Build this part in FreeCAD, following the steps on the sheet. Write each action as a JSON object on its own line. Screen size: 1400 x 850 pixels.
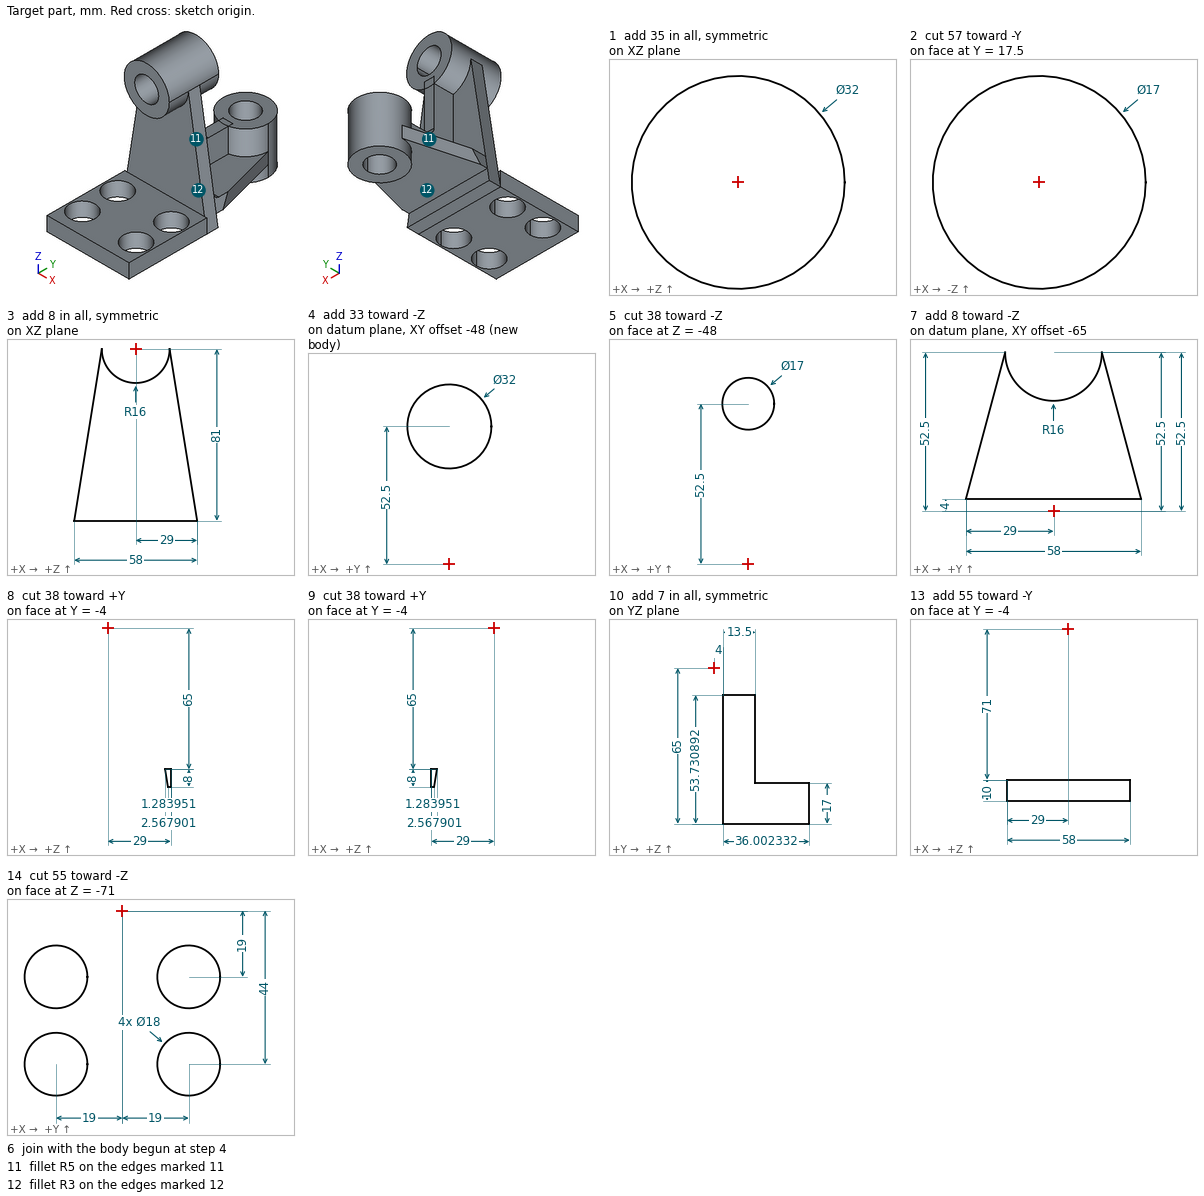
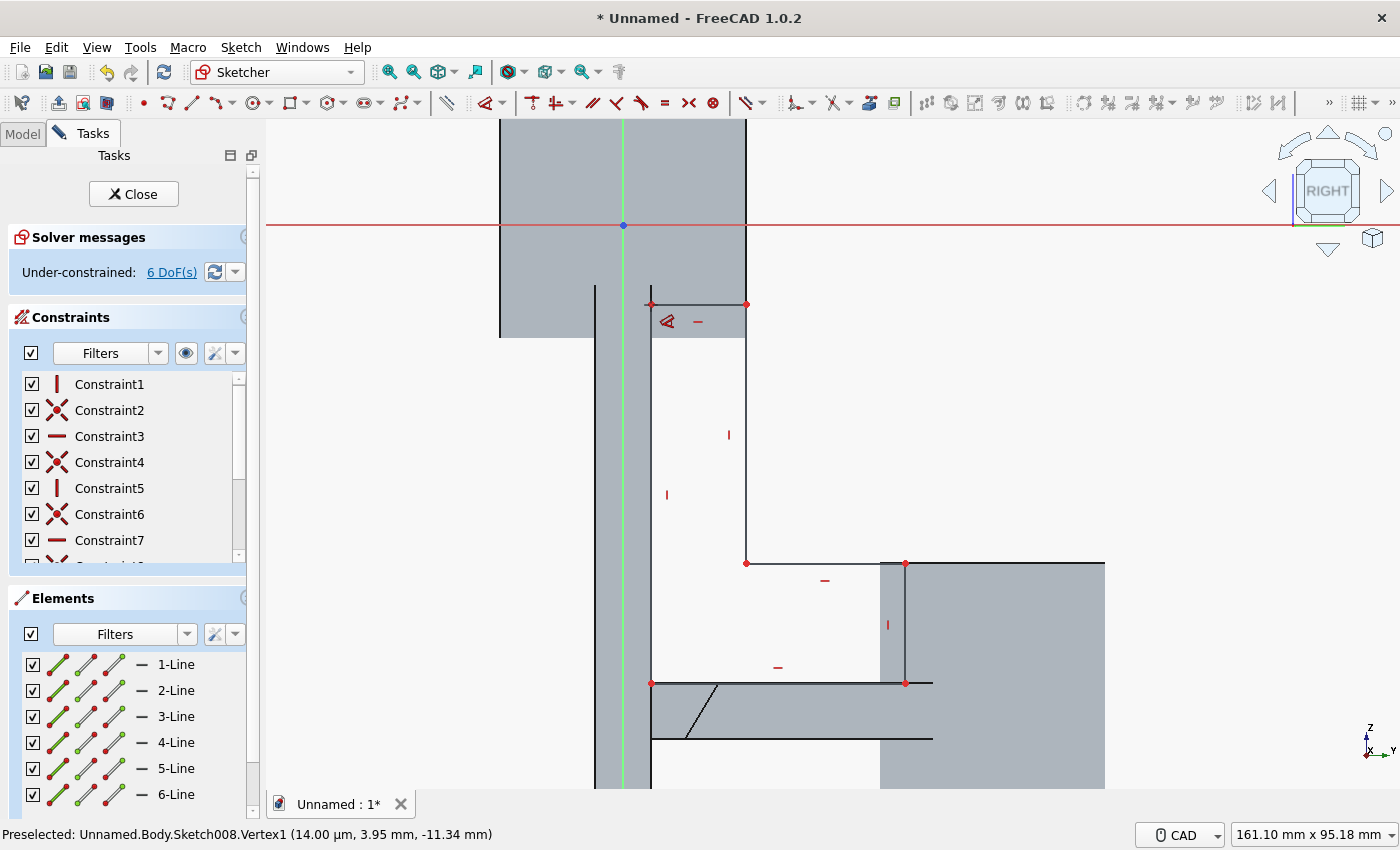
{"action": "left_click", "coordinate": [905, 648]}
{"action": "left_click", "coordinate": [939, 624]}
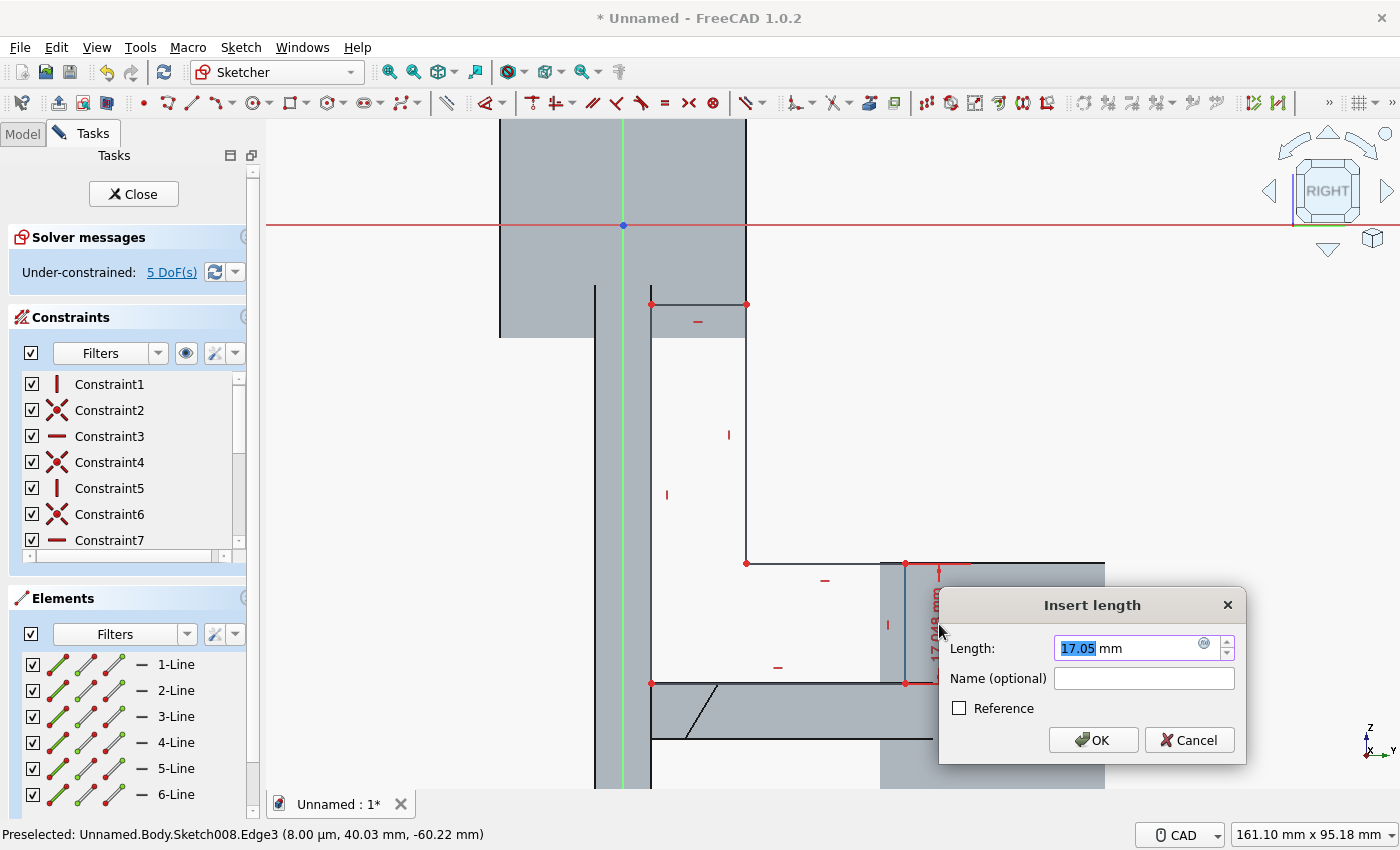
{"action": "type", "text": "17"}
{"action": "key", "text": "Return"}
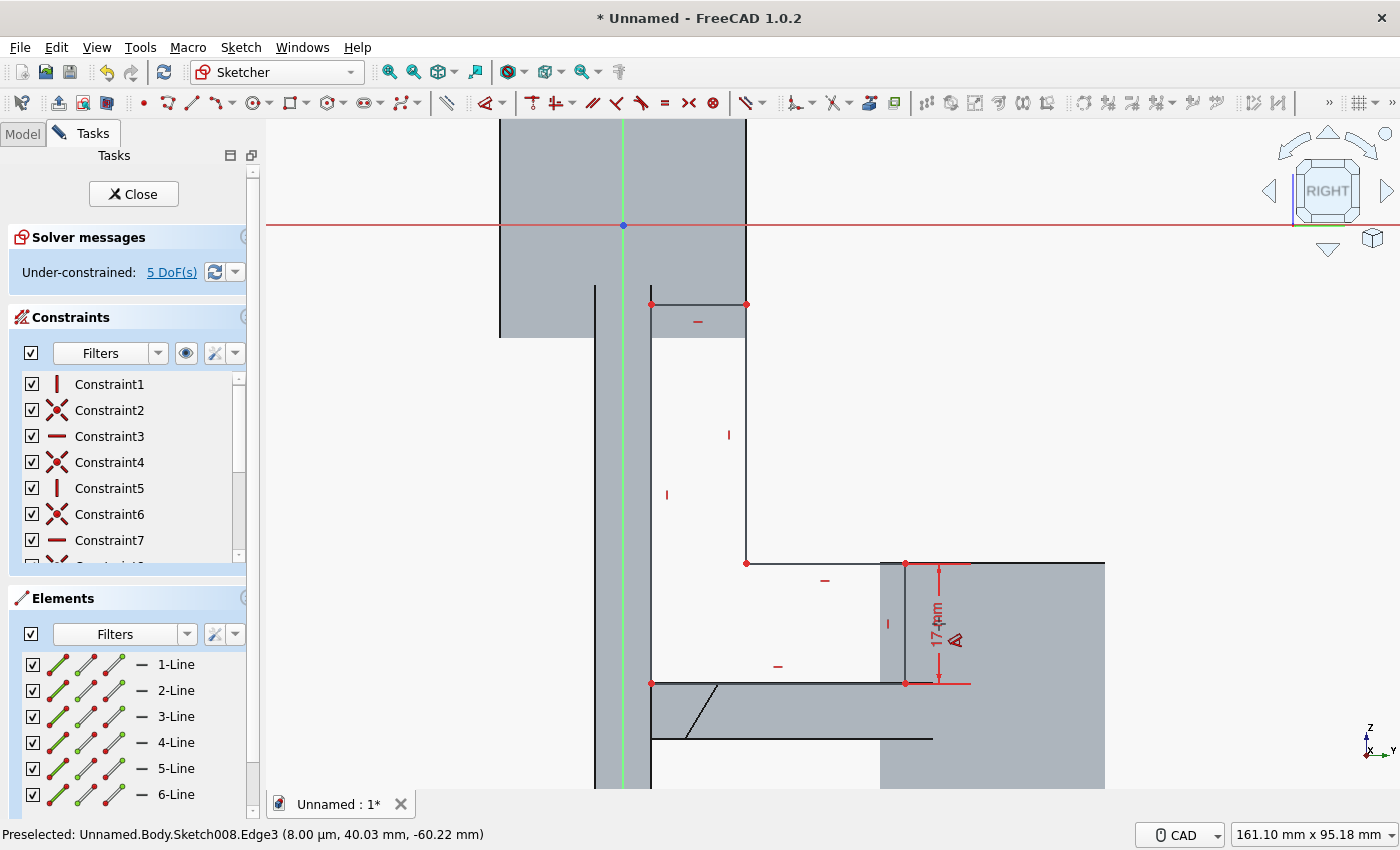
{"action": "scroll", "coordinate": [651, 305], "scroll_direction": "up", "scroll_amount": 2}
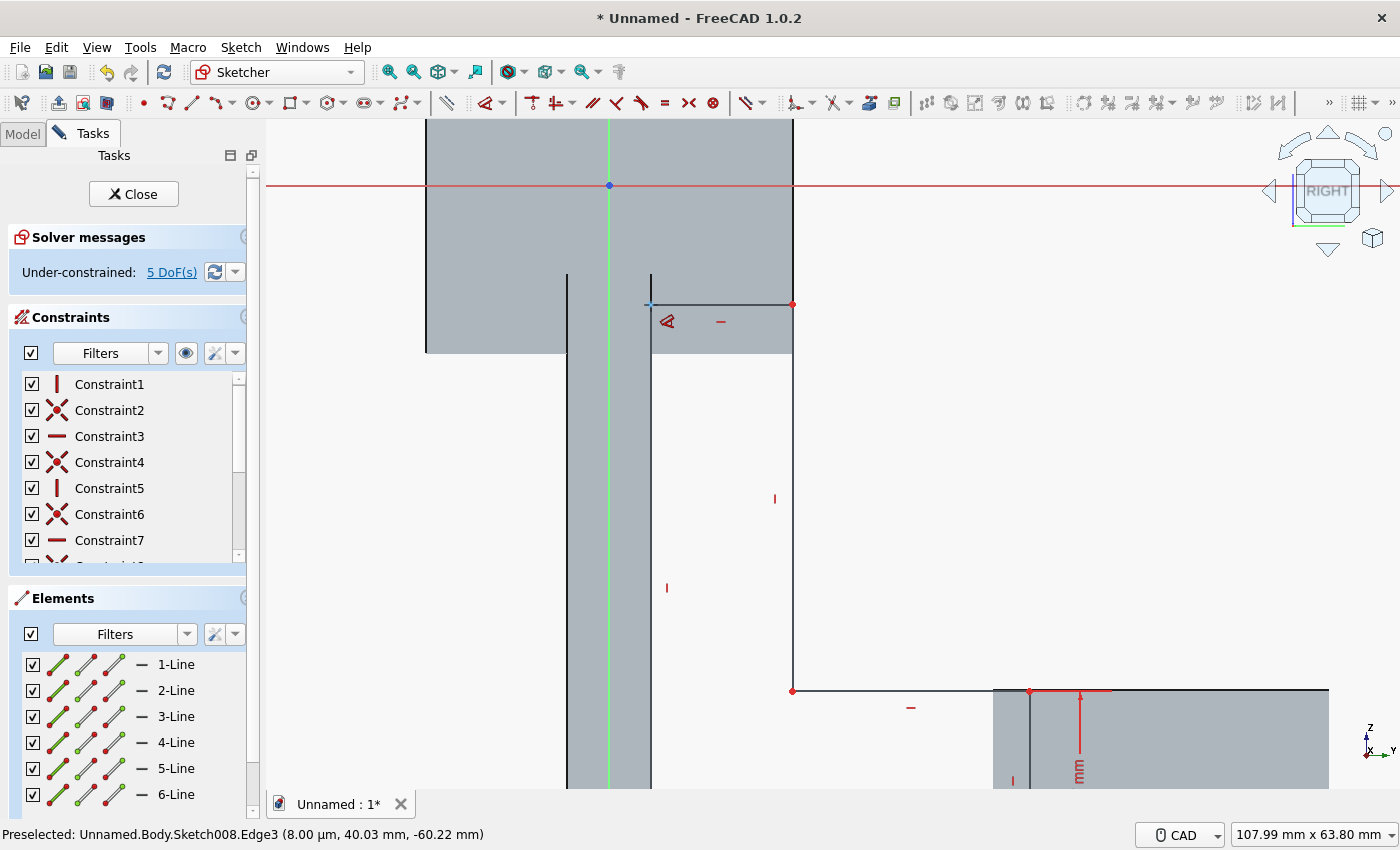
{"action": "left_click", "coordinate": [651, 305]}
{"action": "left_click", "coordinate": [630, 152]}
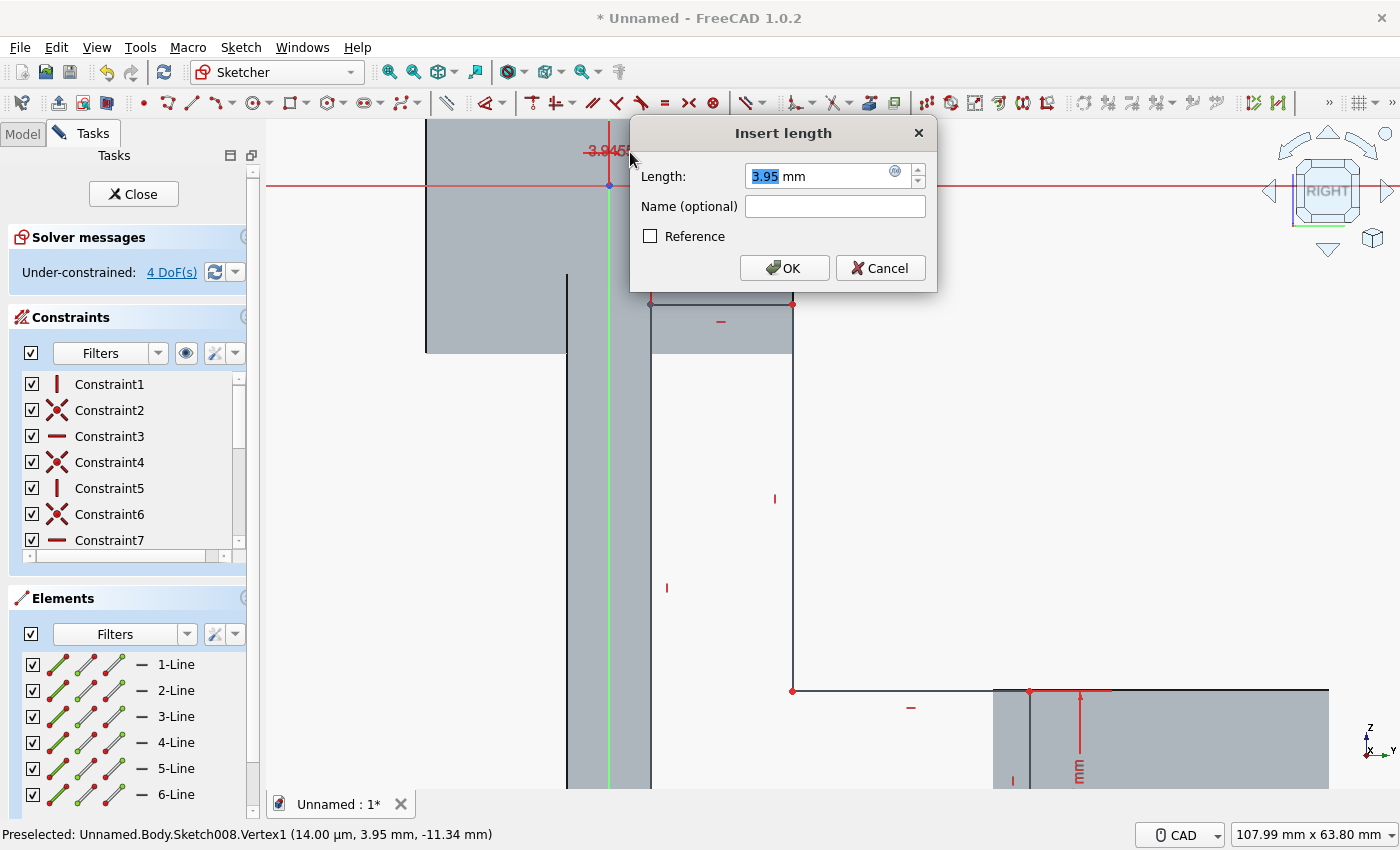
{"action": "type", "text": "4"}
{"action": "key", "text": "Return"}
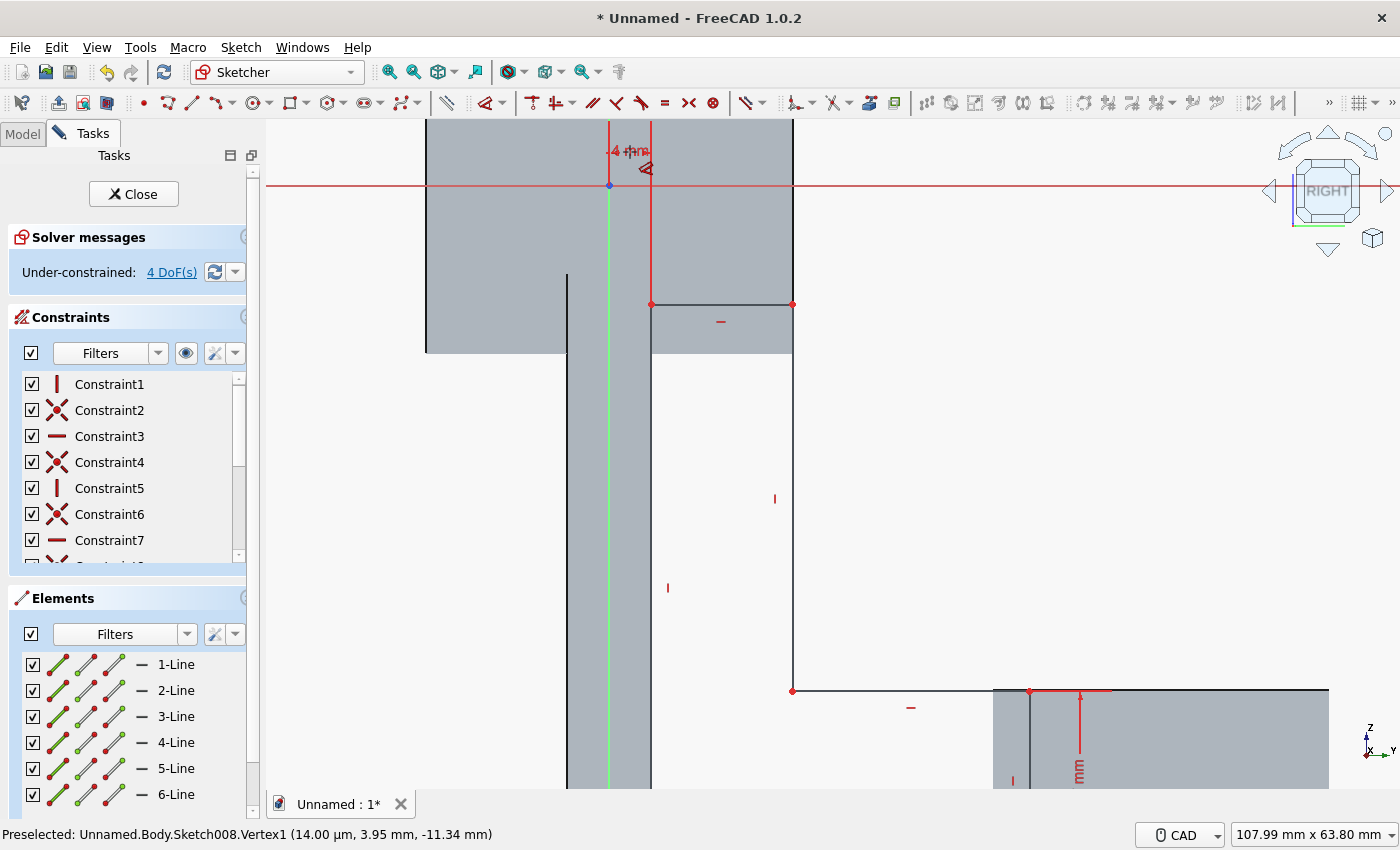
{"action": "scroll", "coordinate": [653, 306], "scroll_direction": "down", "scroll_amount": 2}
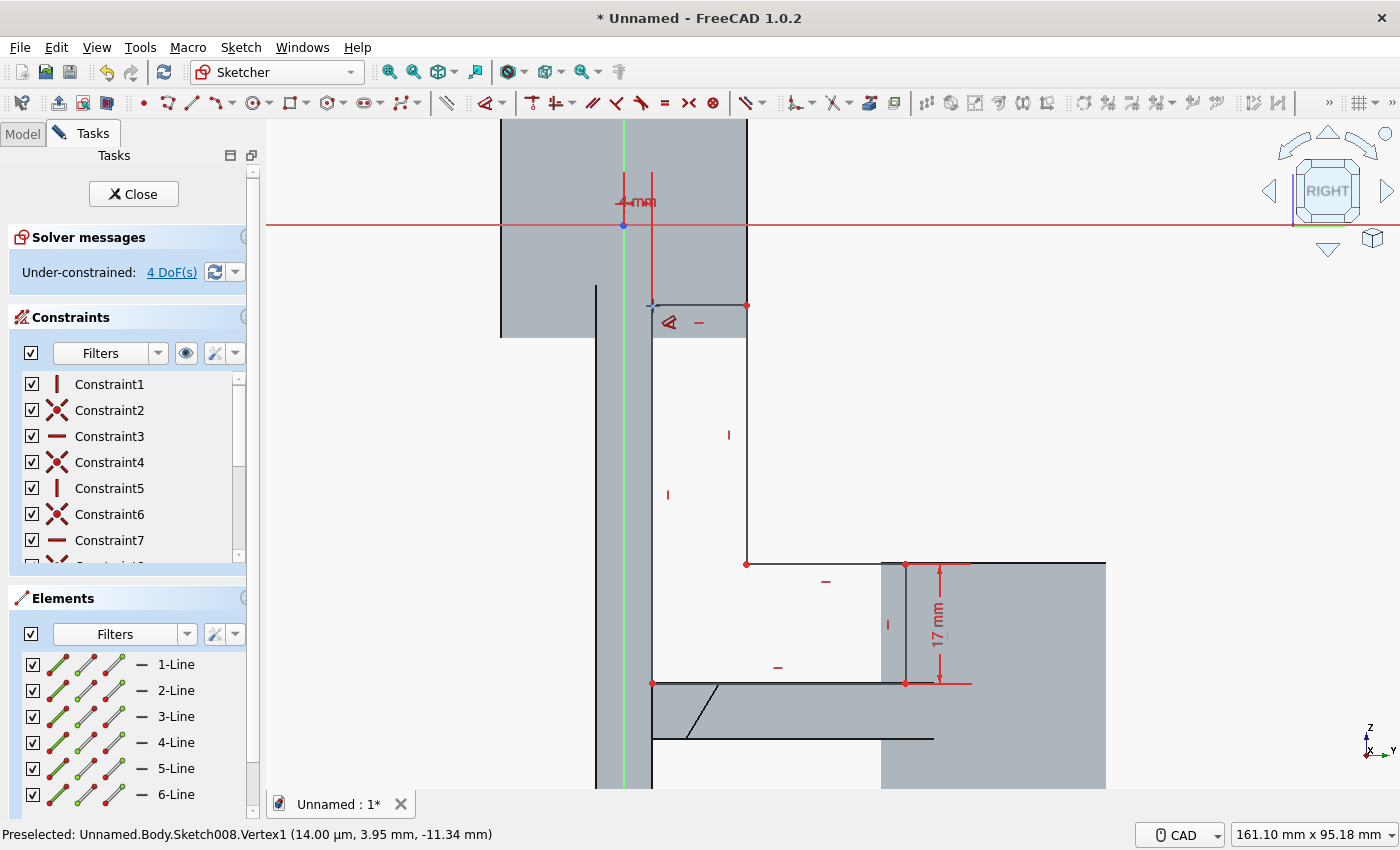
{"action": "left_click", "coordinate": [652, 684]}
{"action": "left_click", "coordinate": [590, 455]}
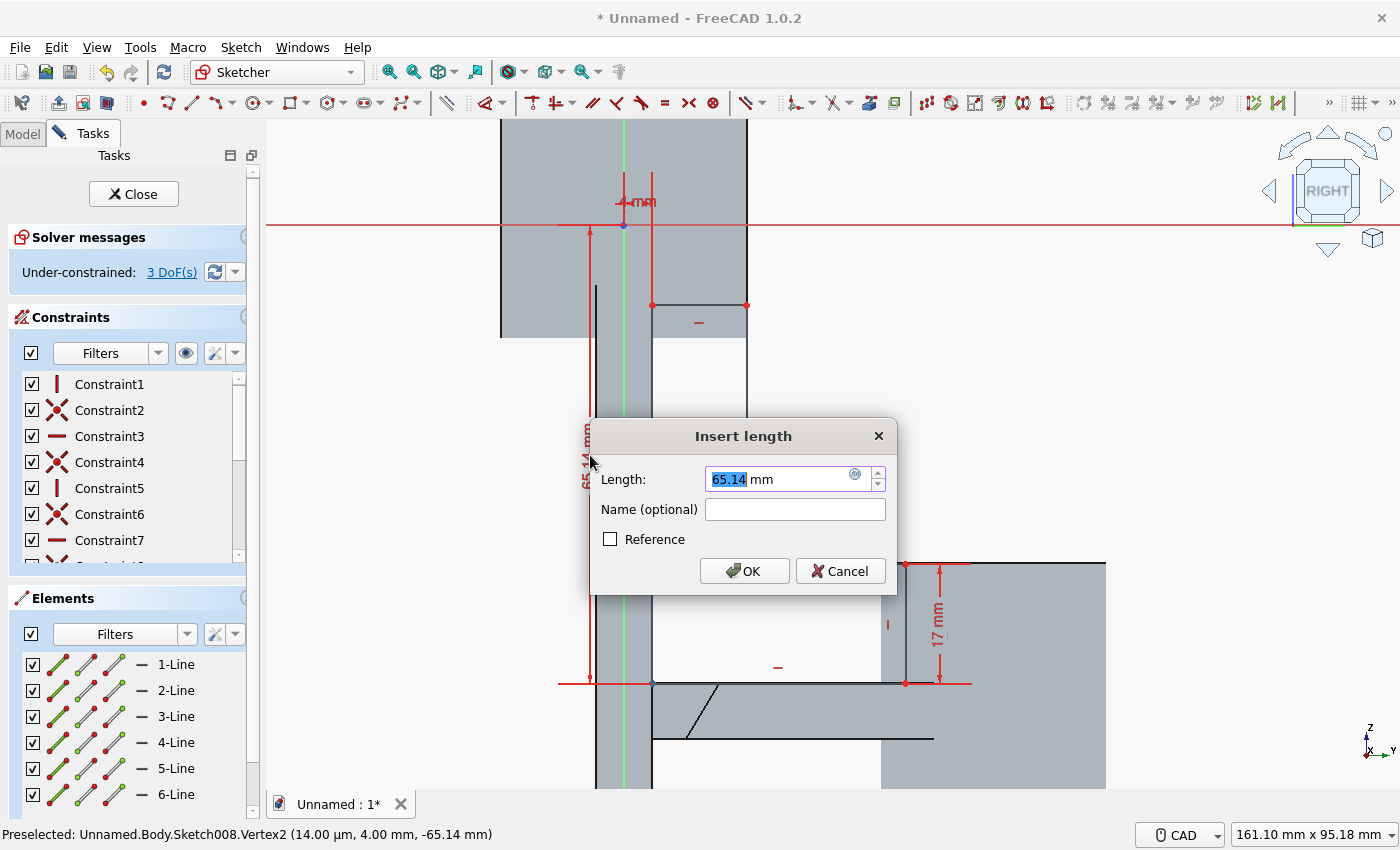
{"action": "type", "text": "65"}
{"action": "key", "text": "Return"}